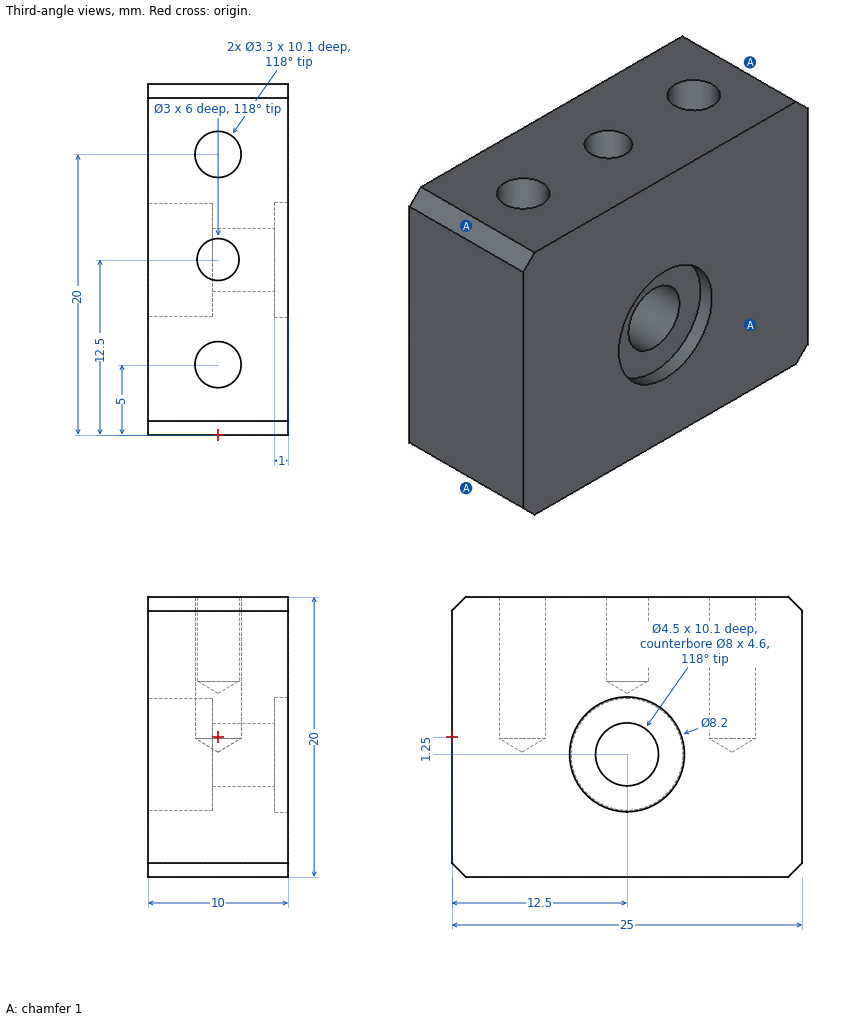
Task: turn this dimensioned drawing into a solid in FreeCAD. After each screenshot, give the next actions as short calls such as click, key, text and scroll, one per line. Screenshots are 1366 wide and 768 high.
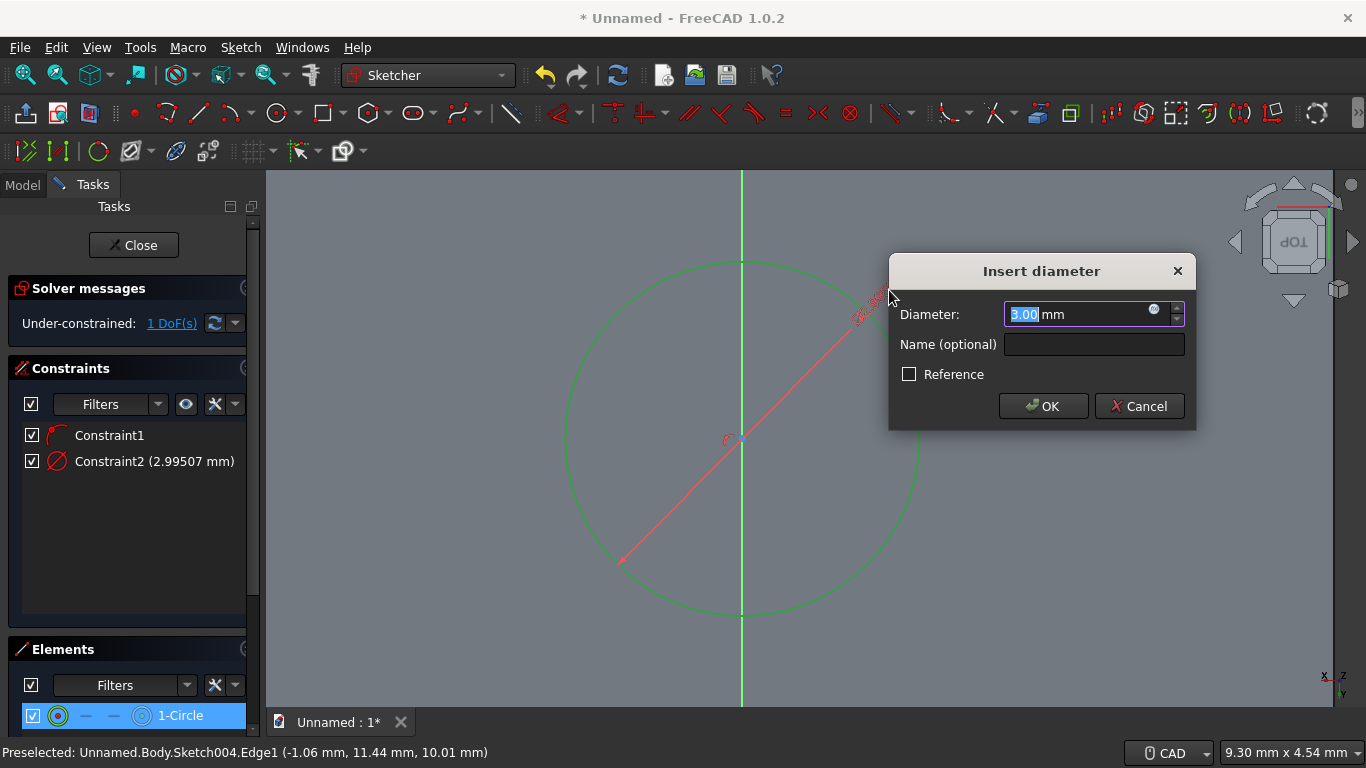
text(3)
key(Return)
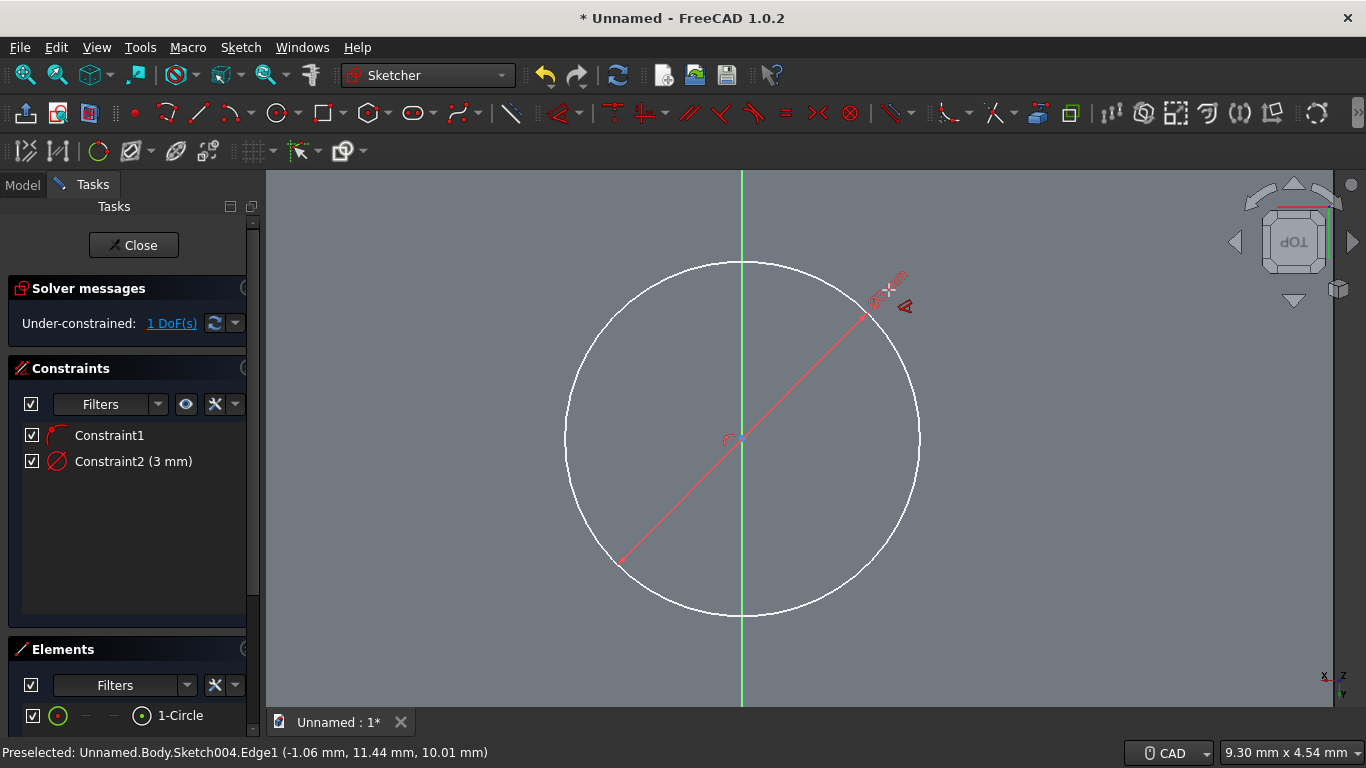
click(742, 439)
click(776, 319)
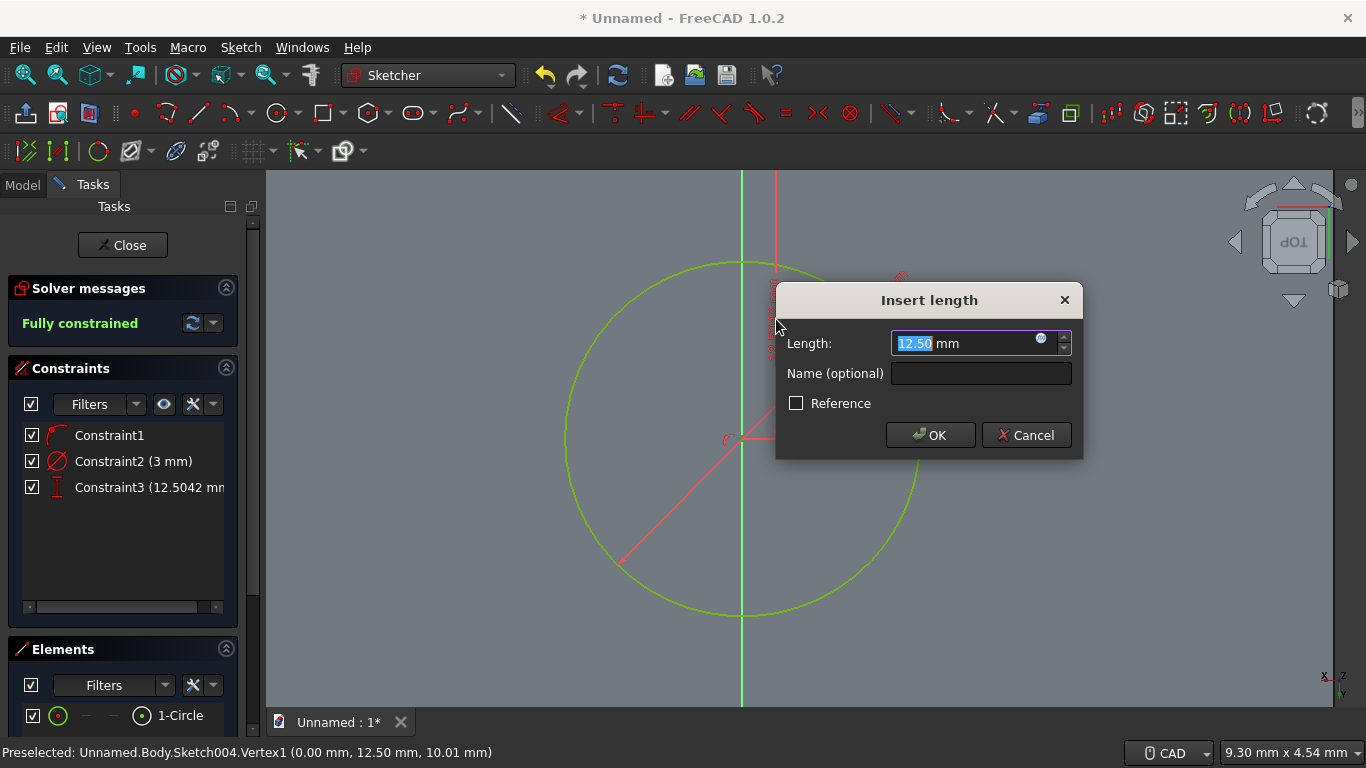
text(12.5)
key(Return)
key(Escape)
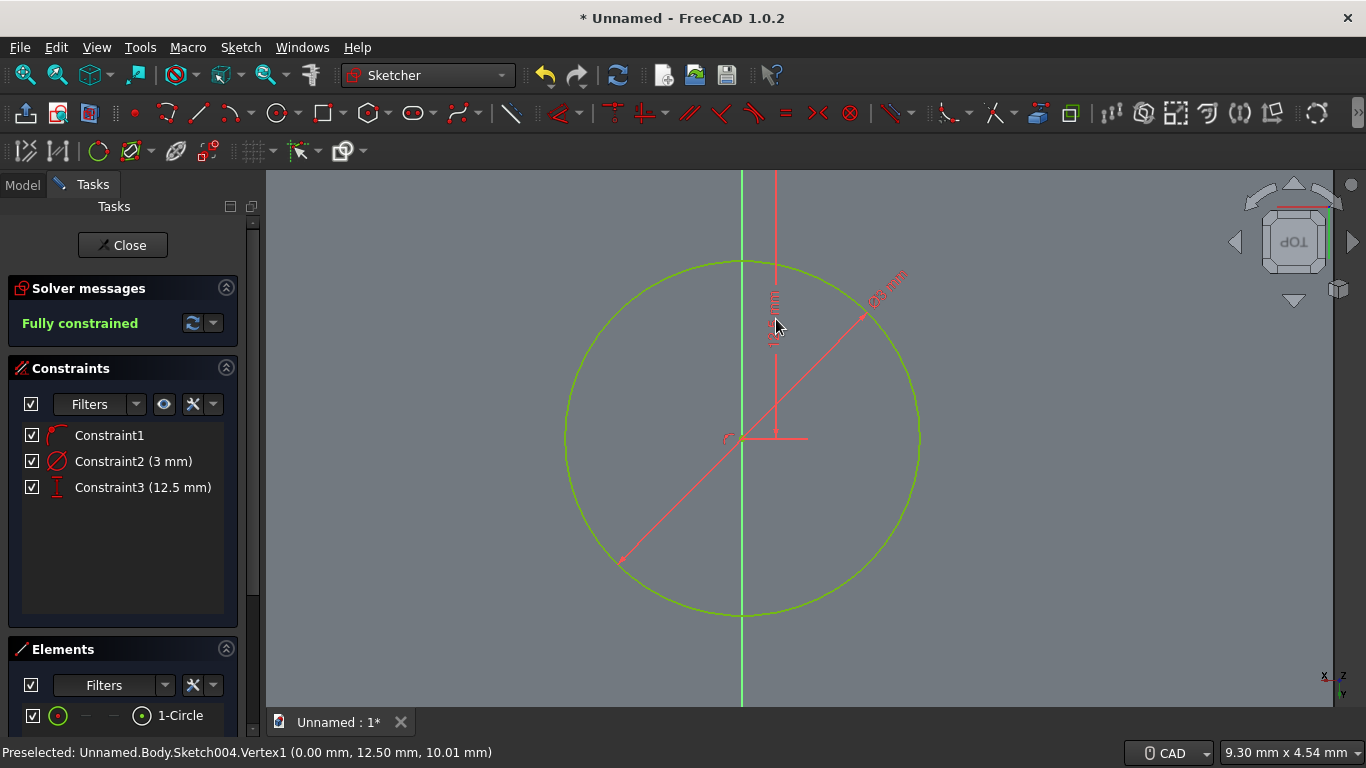
click(123, 245)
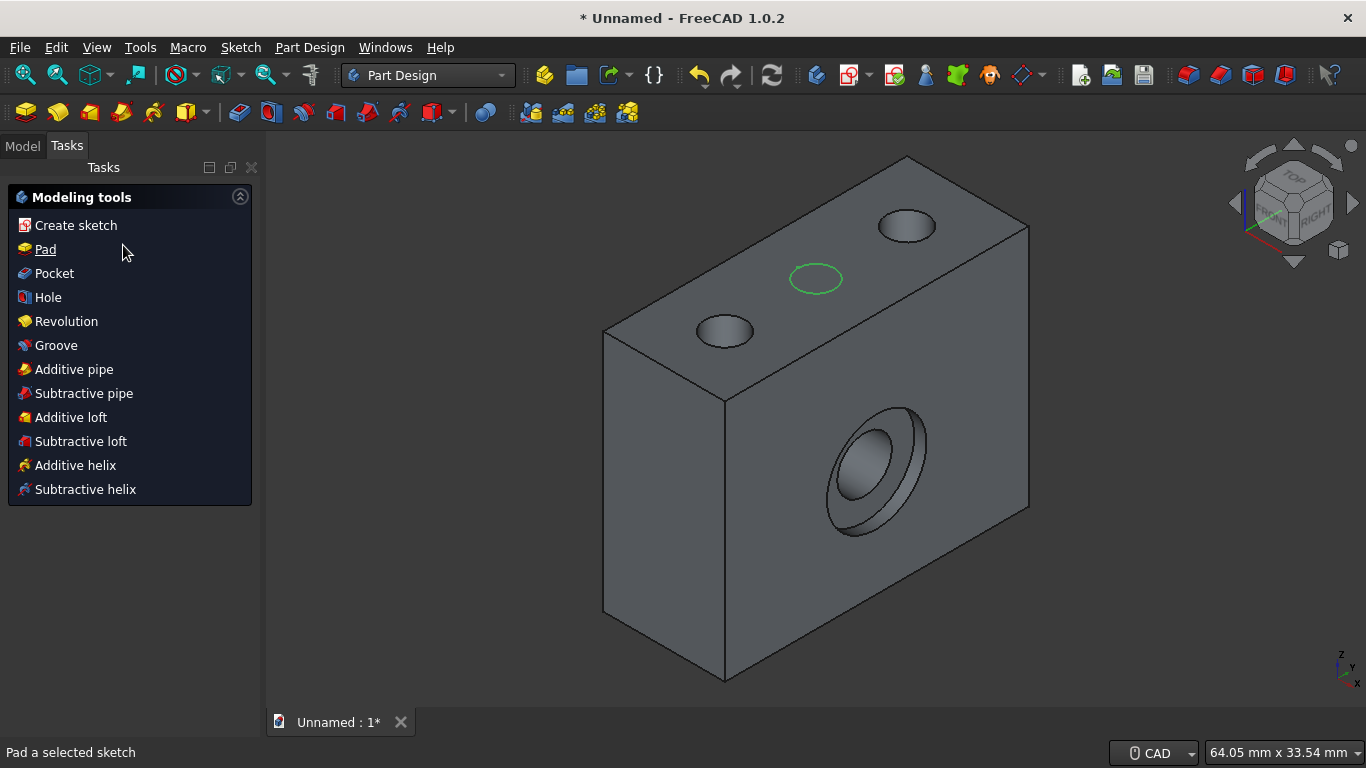
click(272, 112)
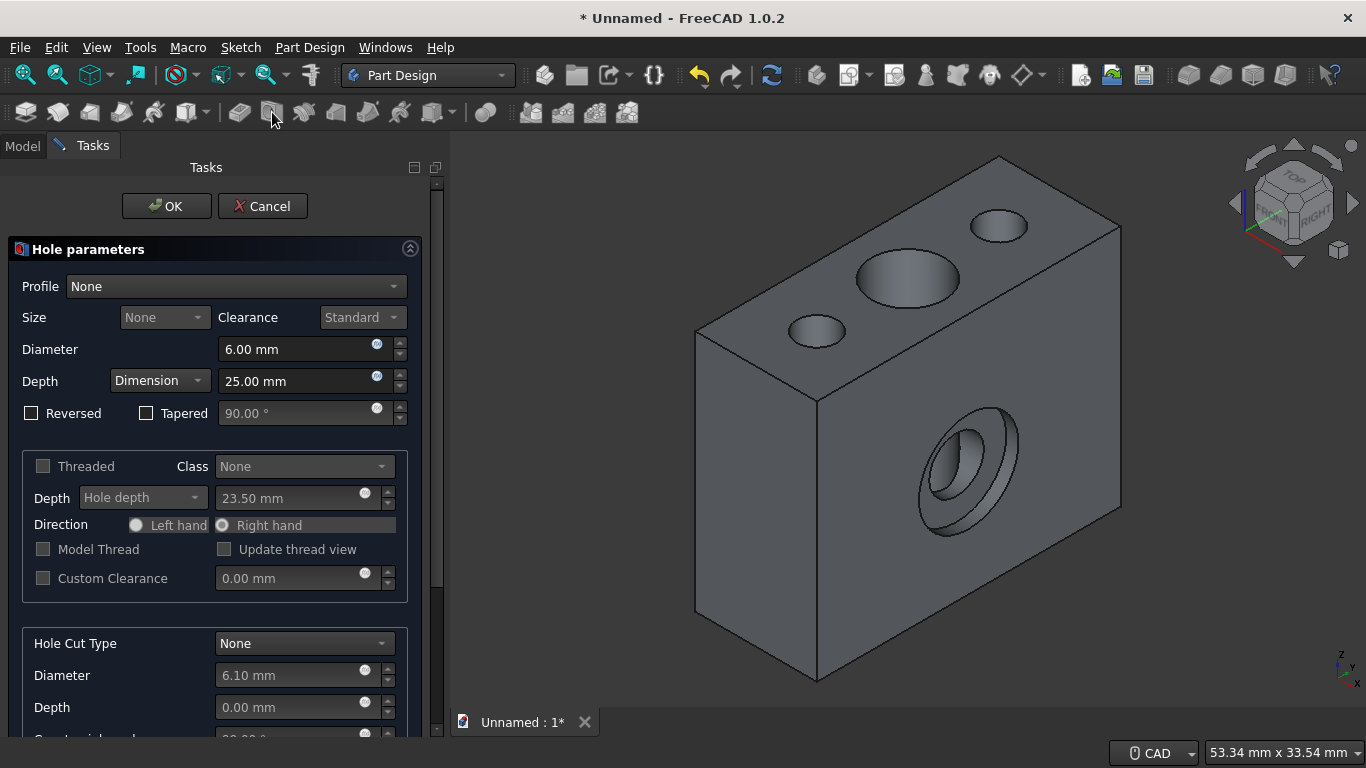
triple_click(305, 349)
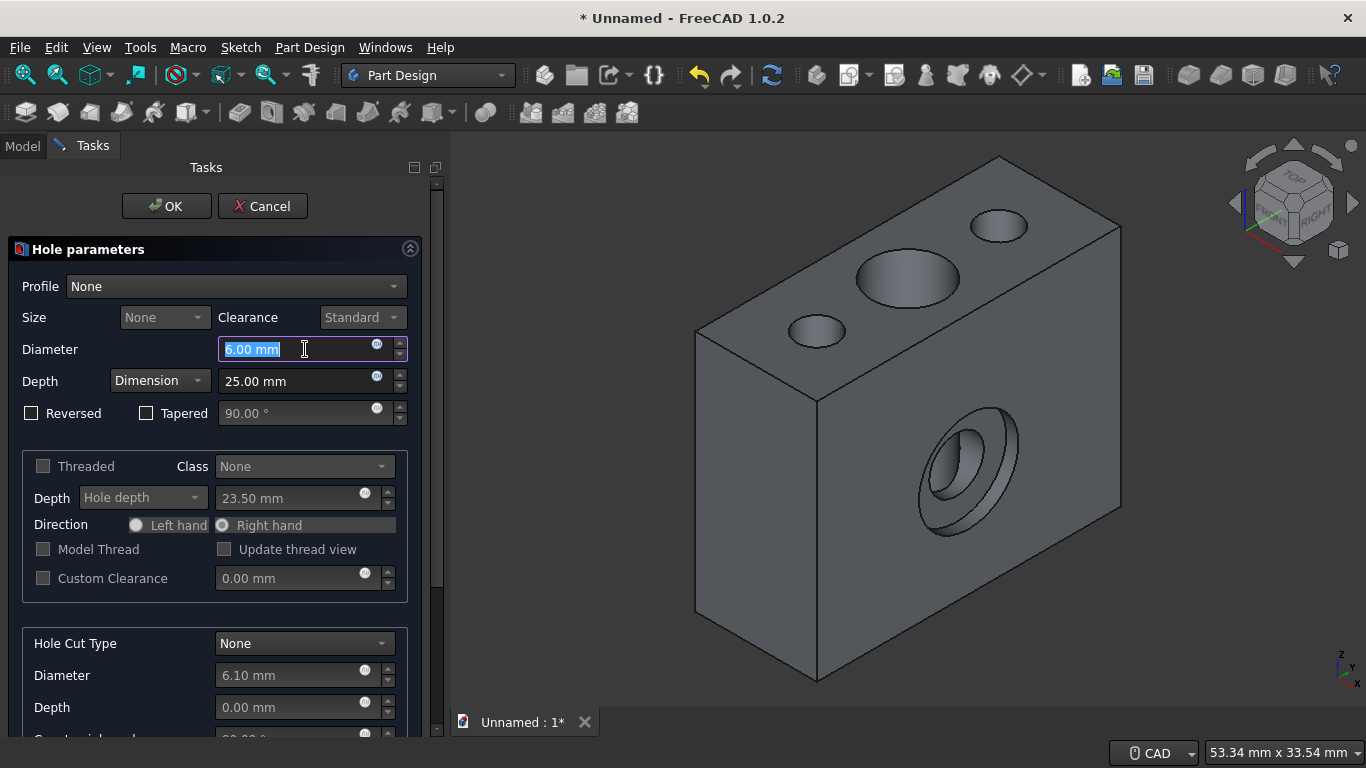
text(3)
key(Tab)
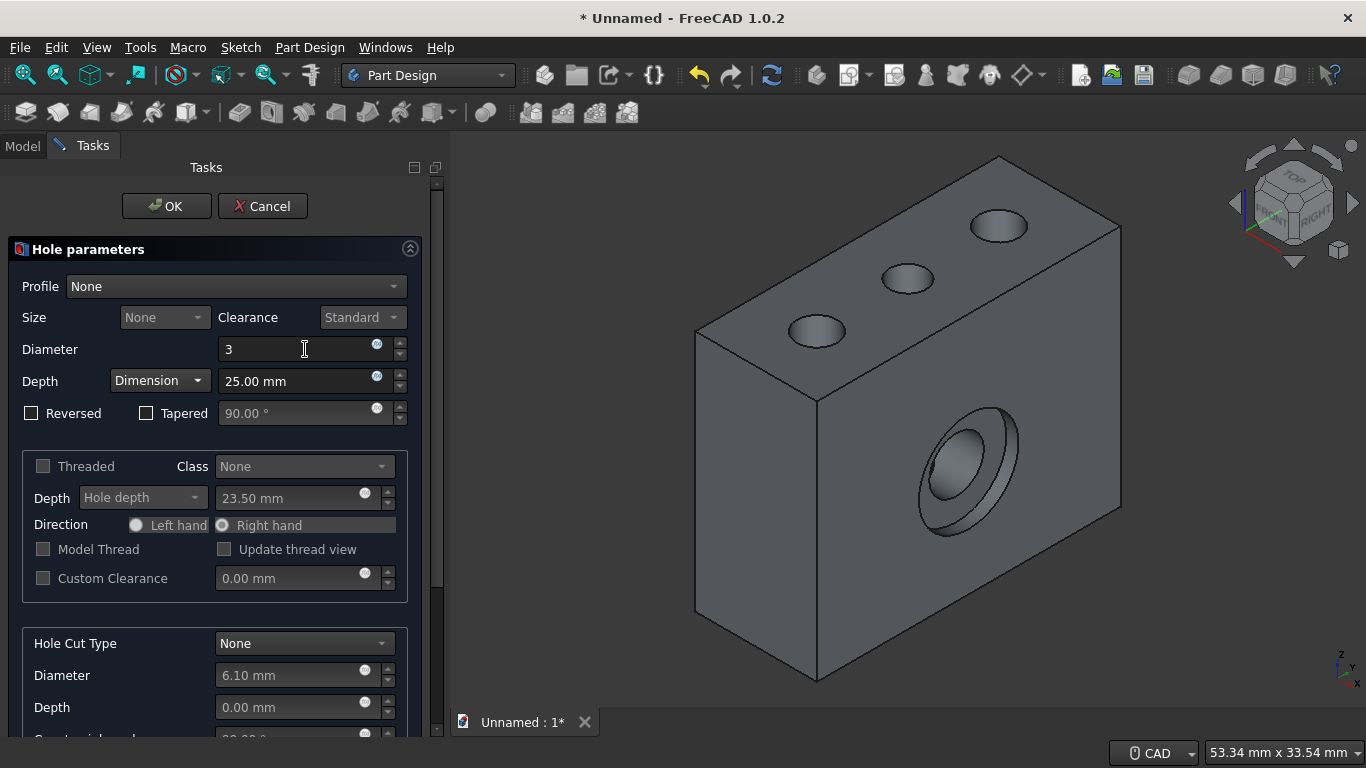
triple_click(305, 381)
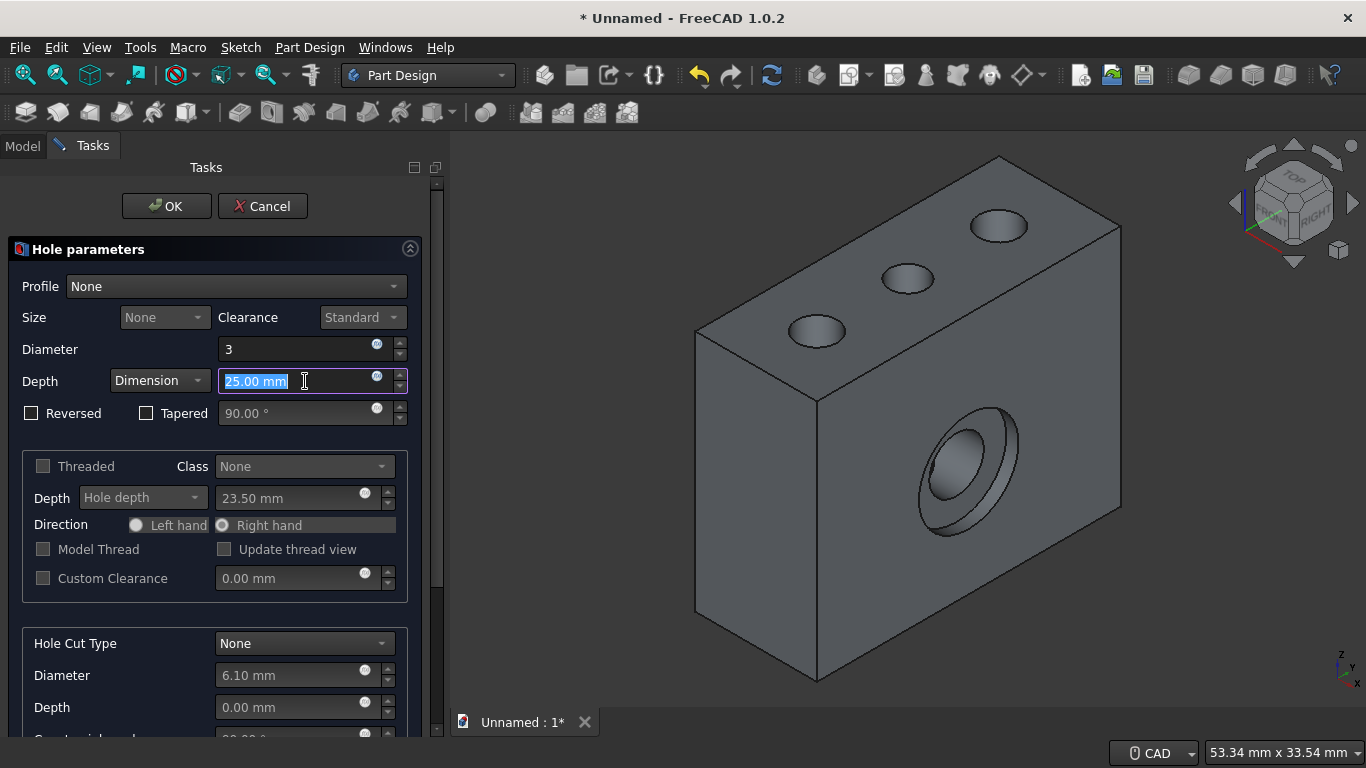
text(6)
key(Tab)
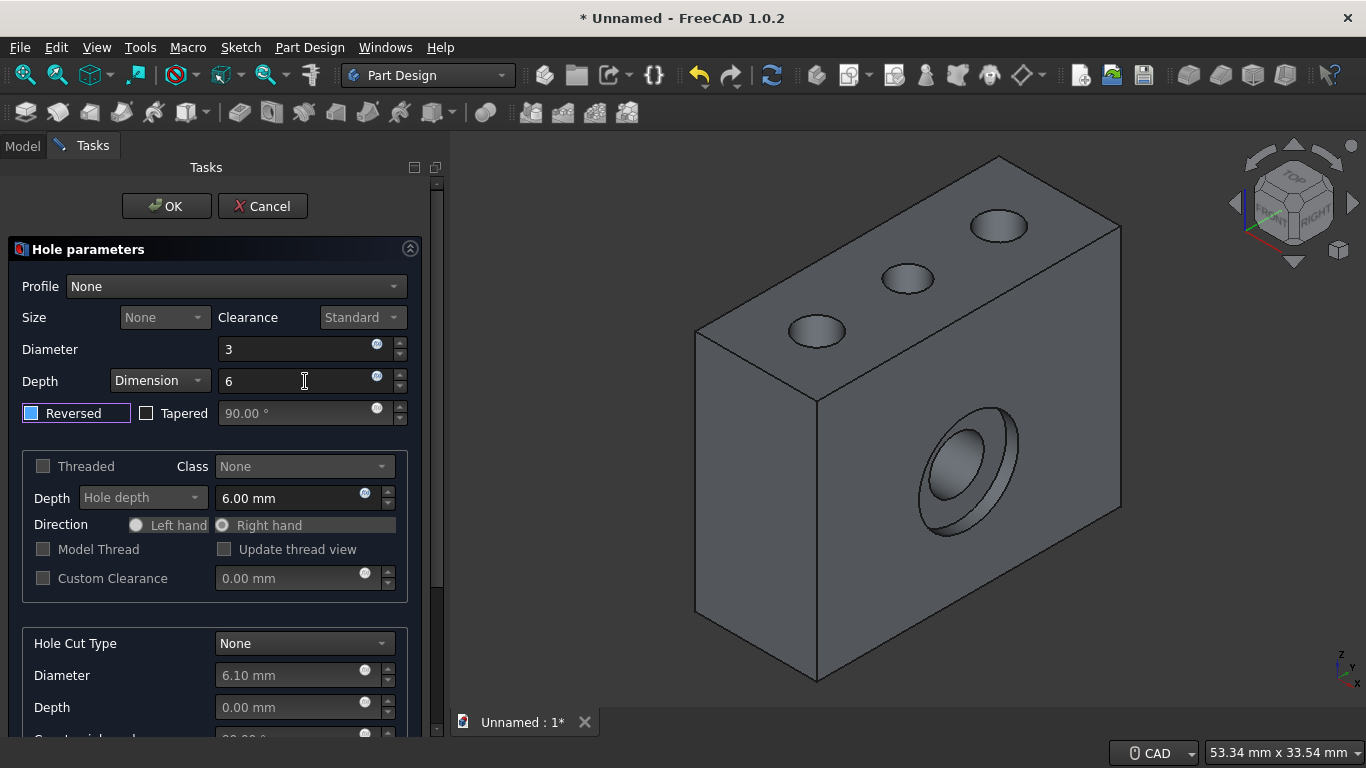
click(167, 206)